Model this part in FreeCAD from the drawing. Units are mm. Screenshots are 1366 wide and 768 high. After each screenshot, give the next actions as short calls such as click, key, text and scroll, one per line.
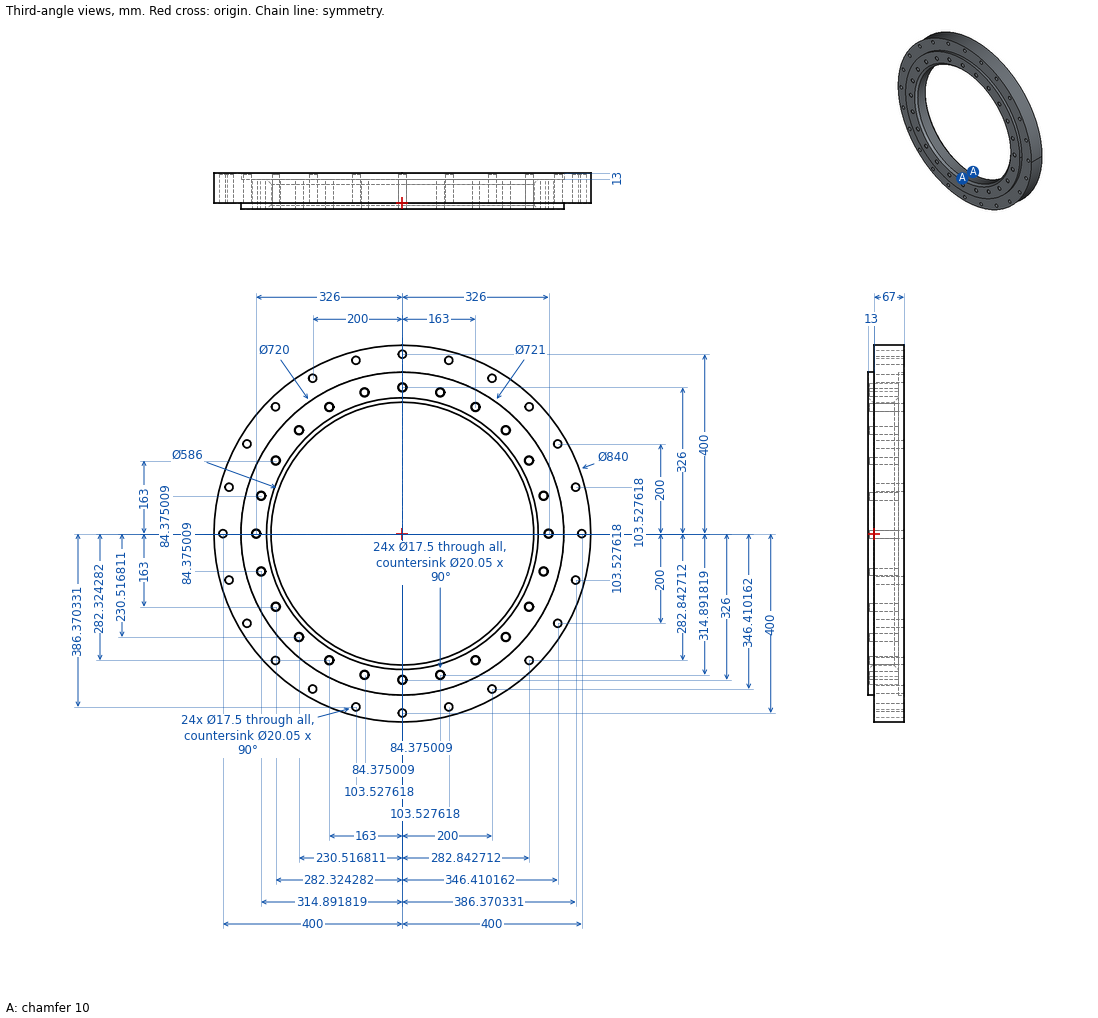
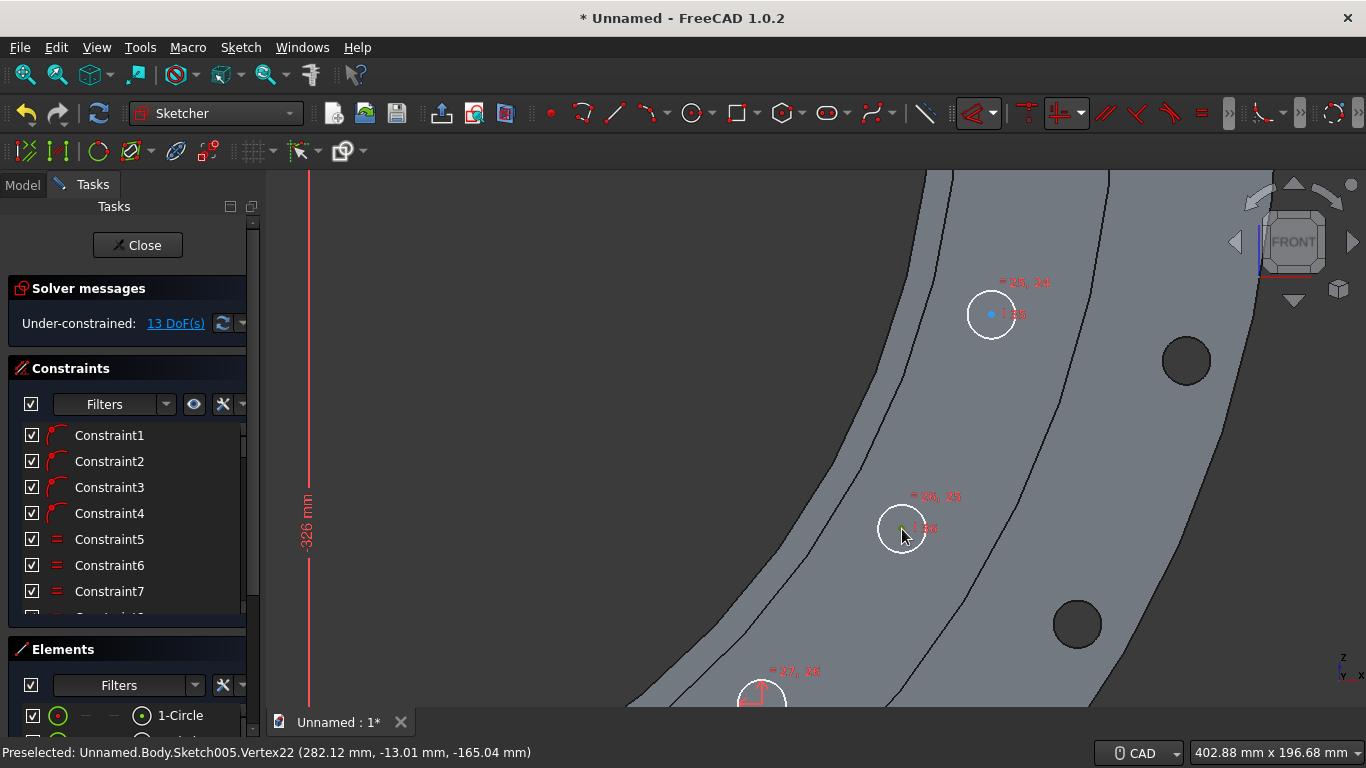
key(i)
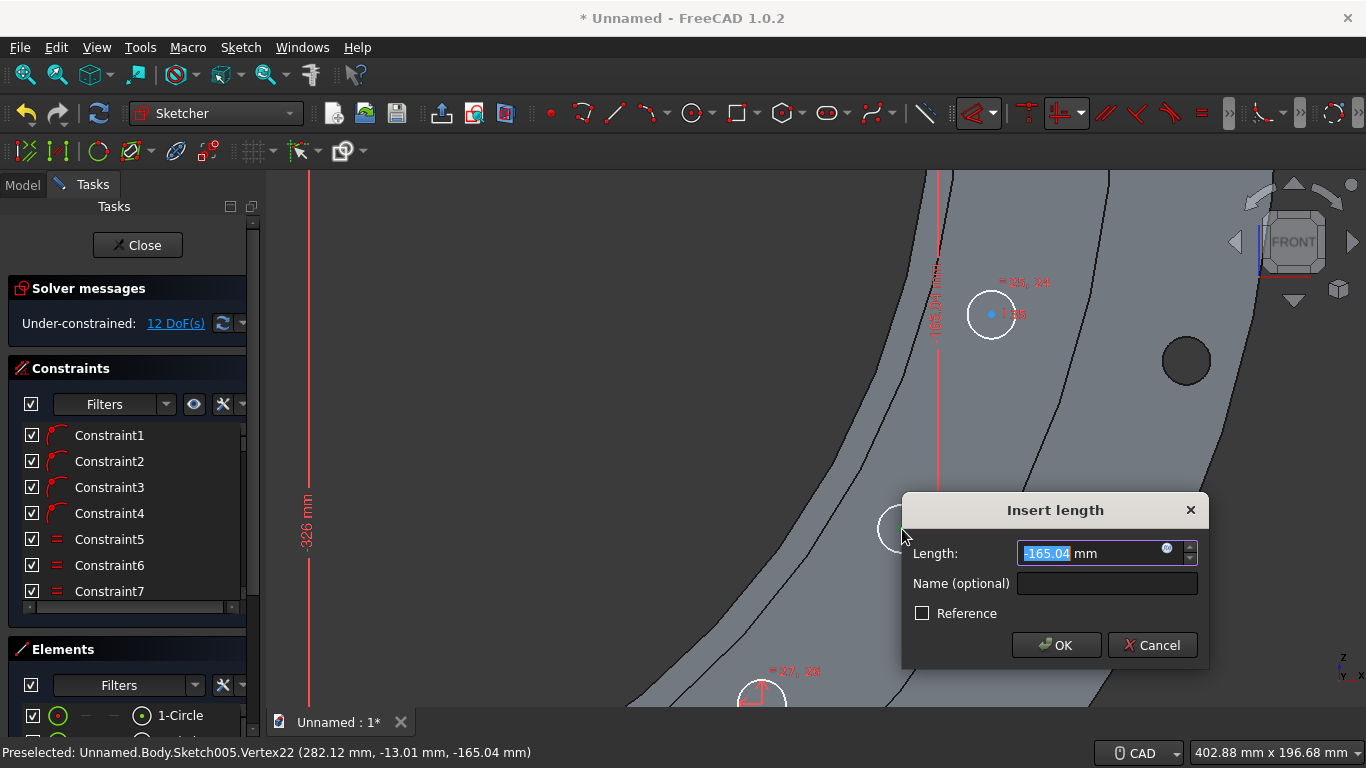
text(-163)
key(Return)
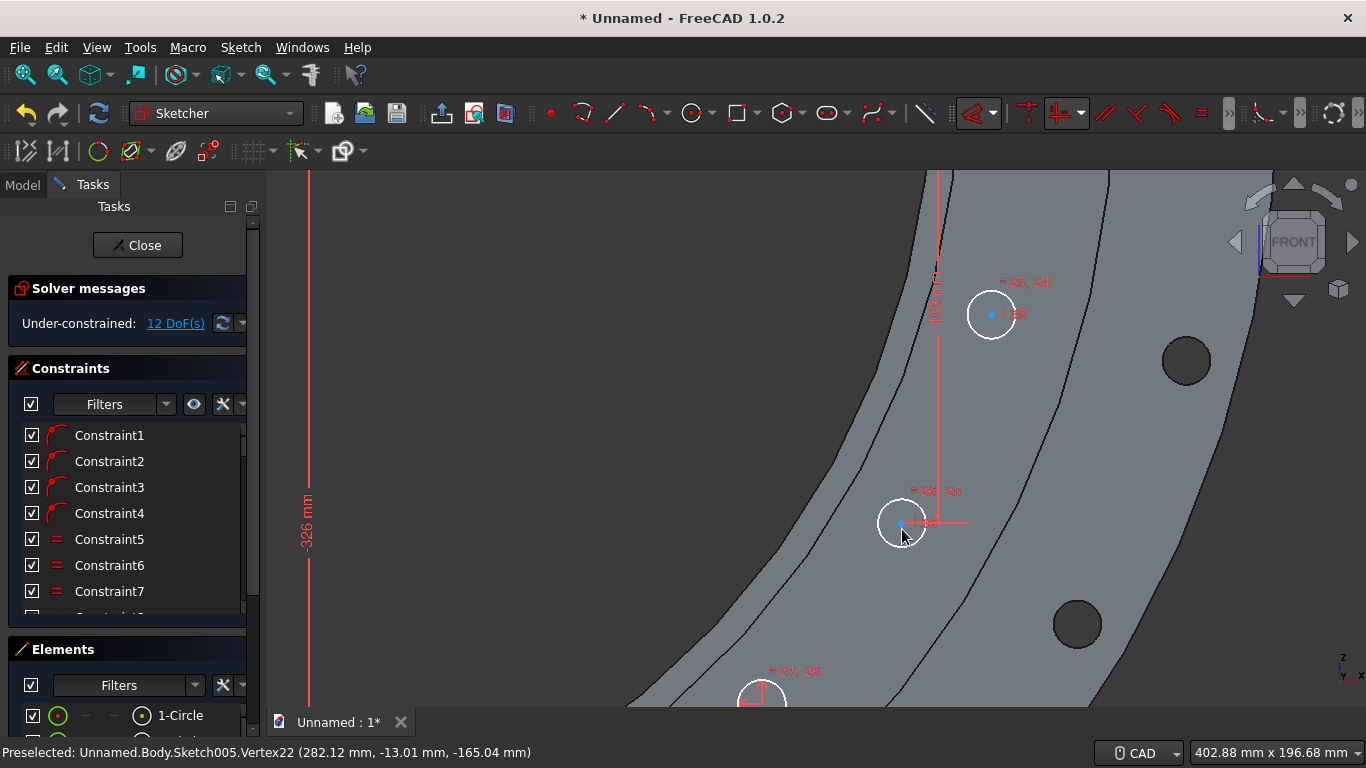
scroll(903, 530, down, 8)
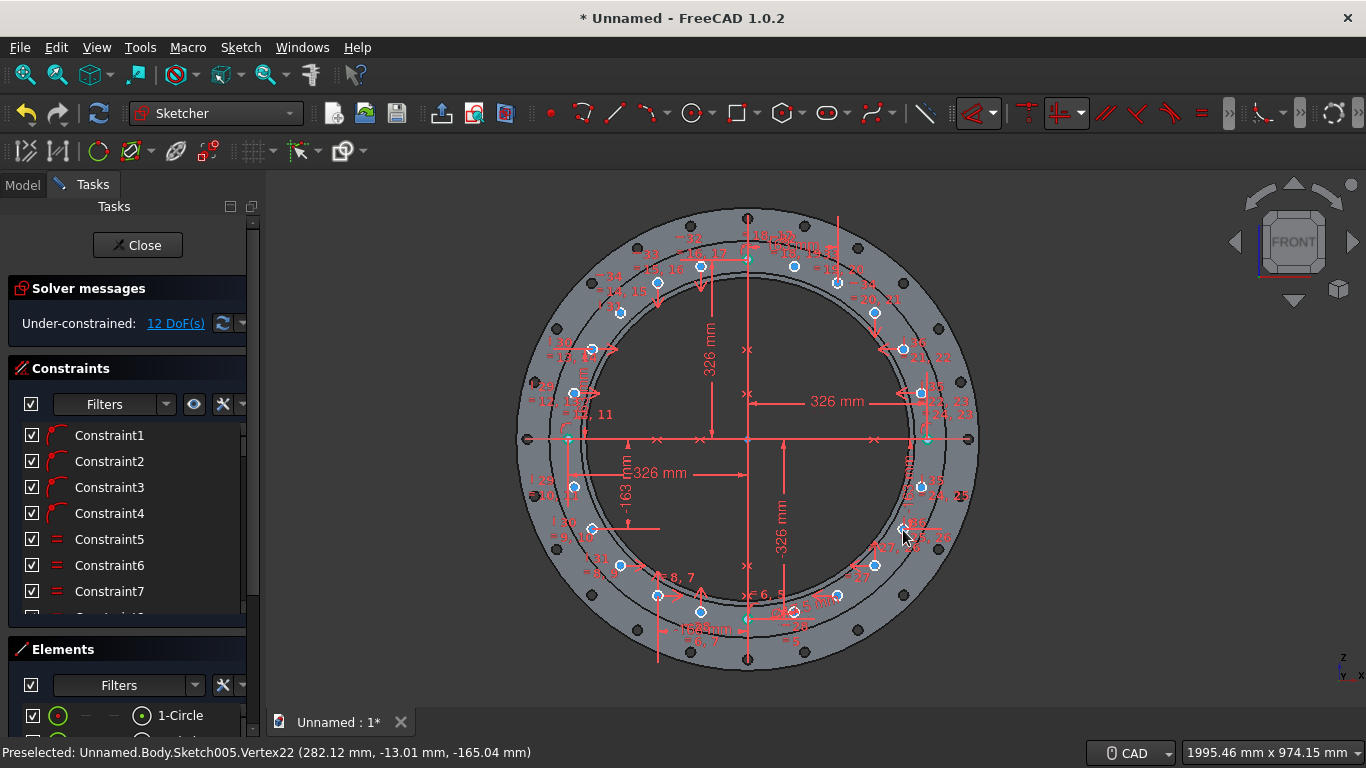
click(794, 612)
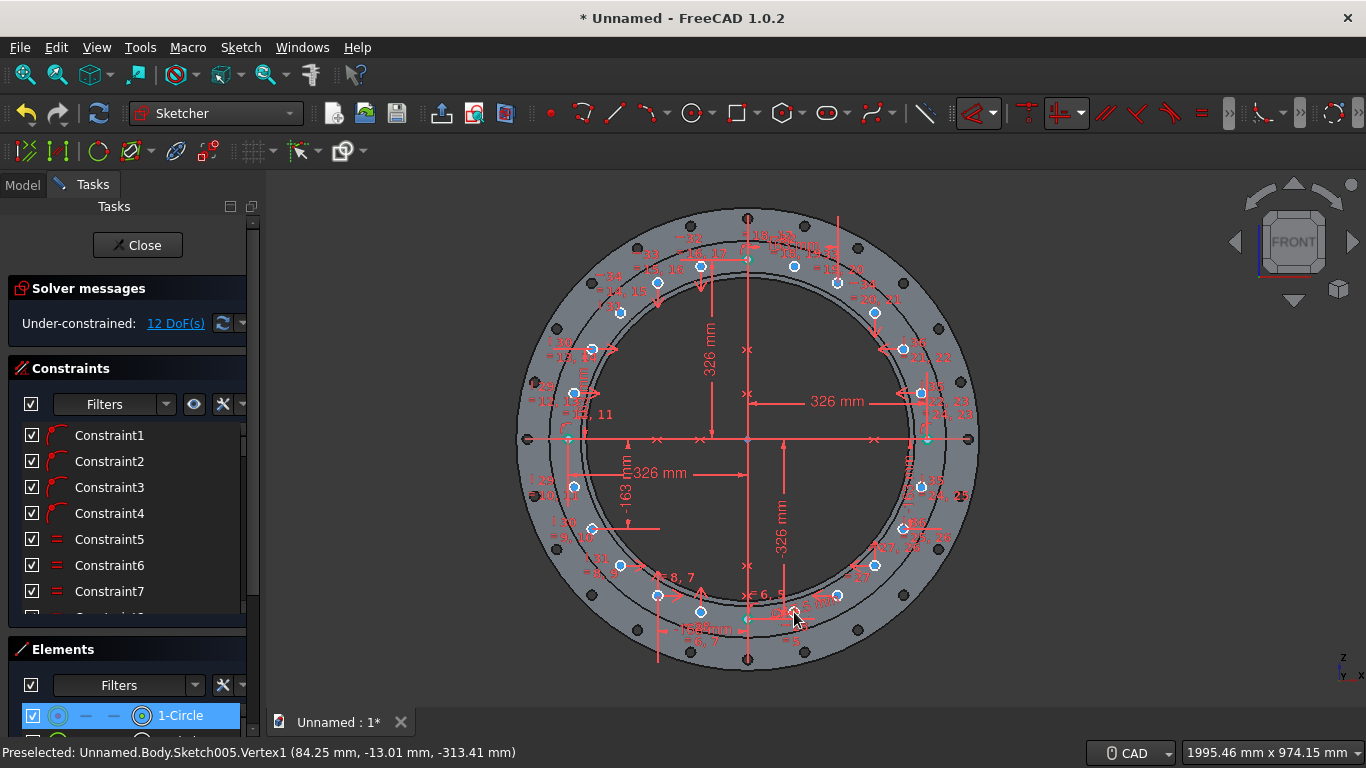
key(l)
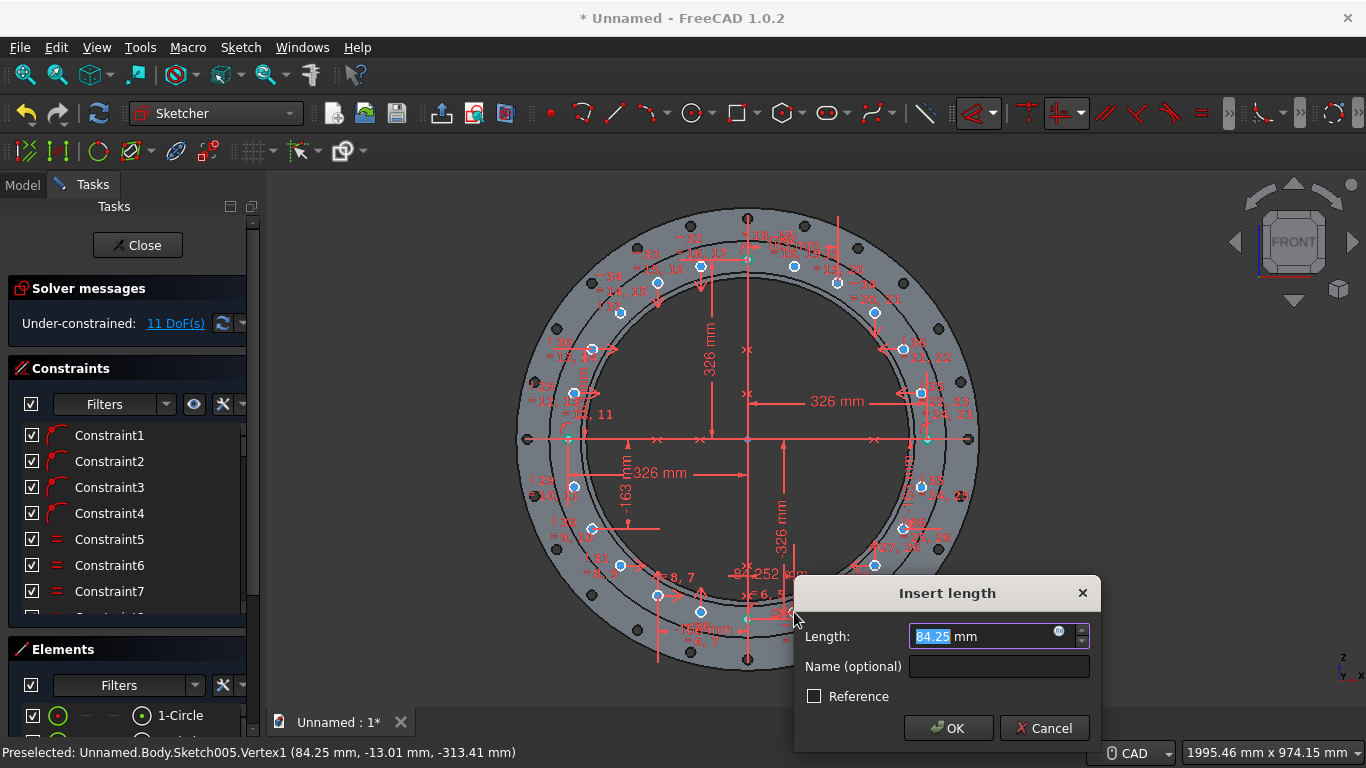
text(84.375009)
key(Return)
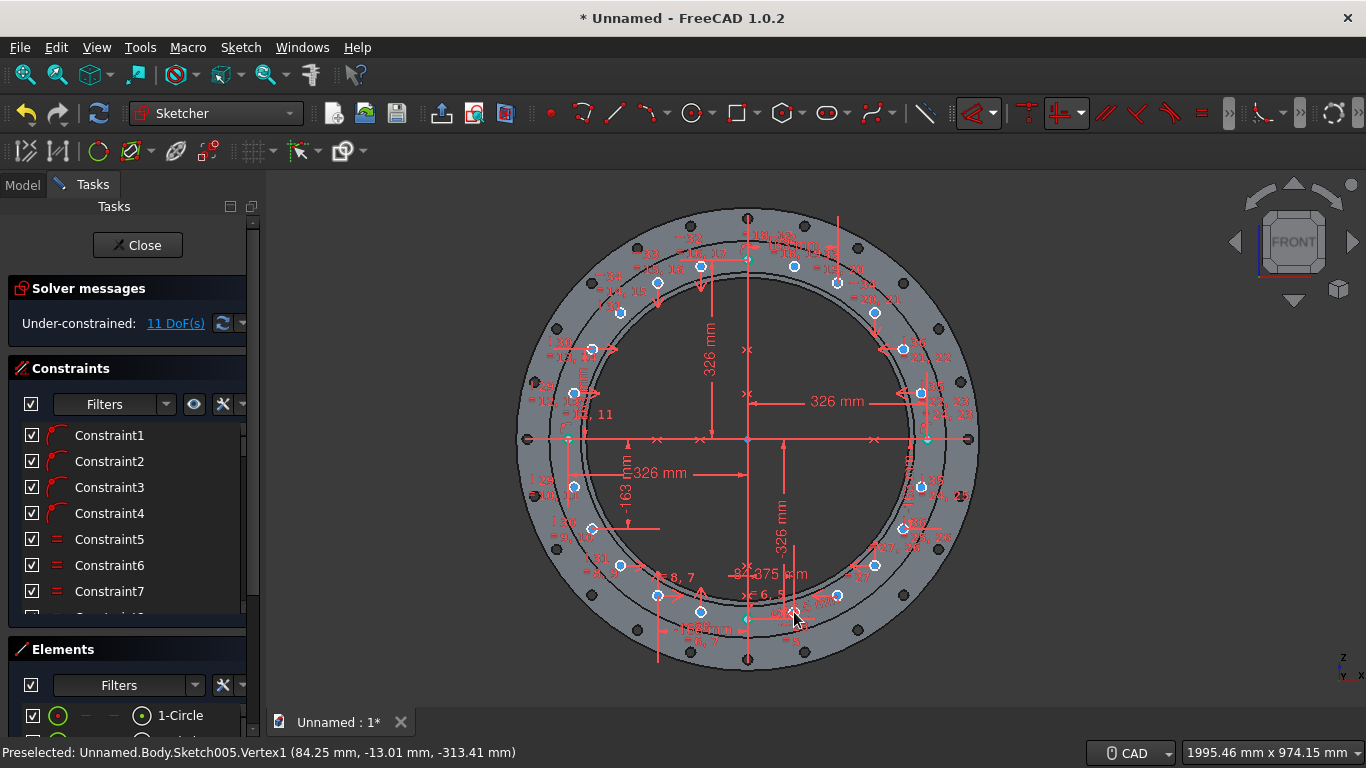
click(701, 612)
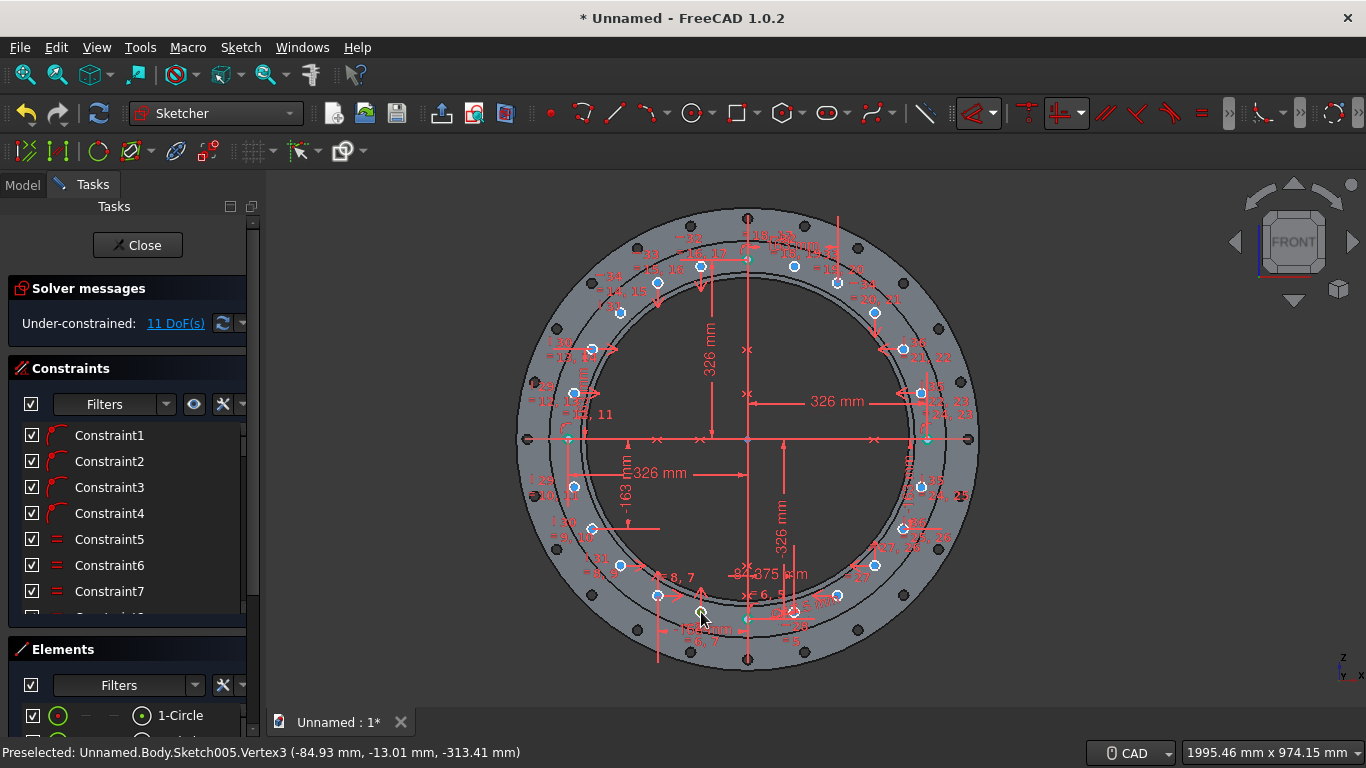
key(l)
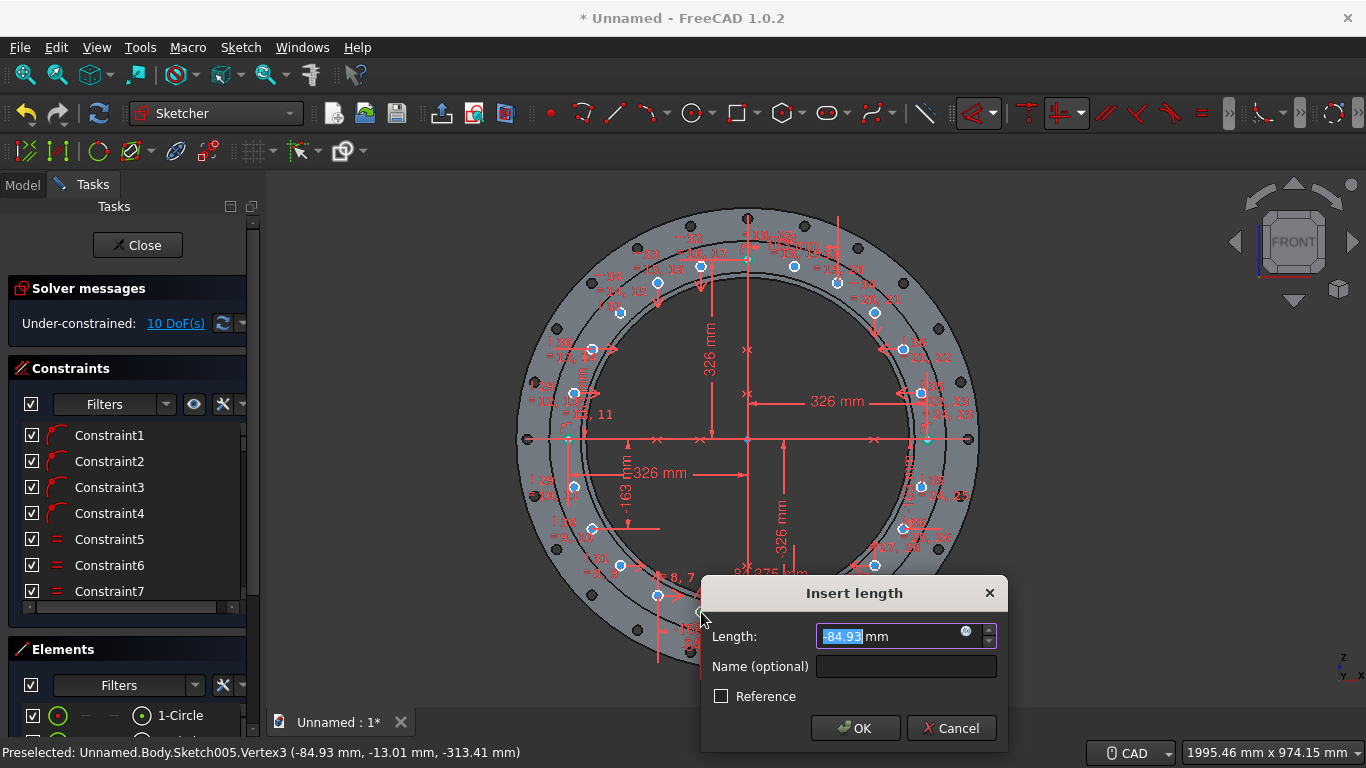
text(-84.375009)
key(Return)